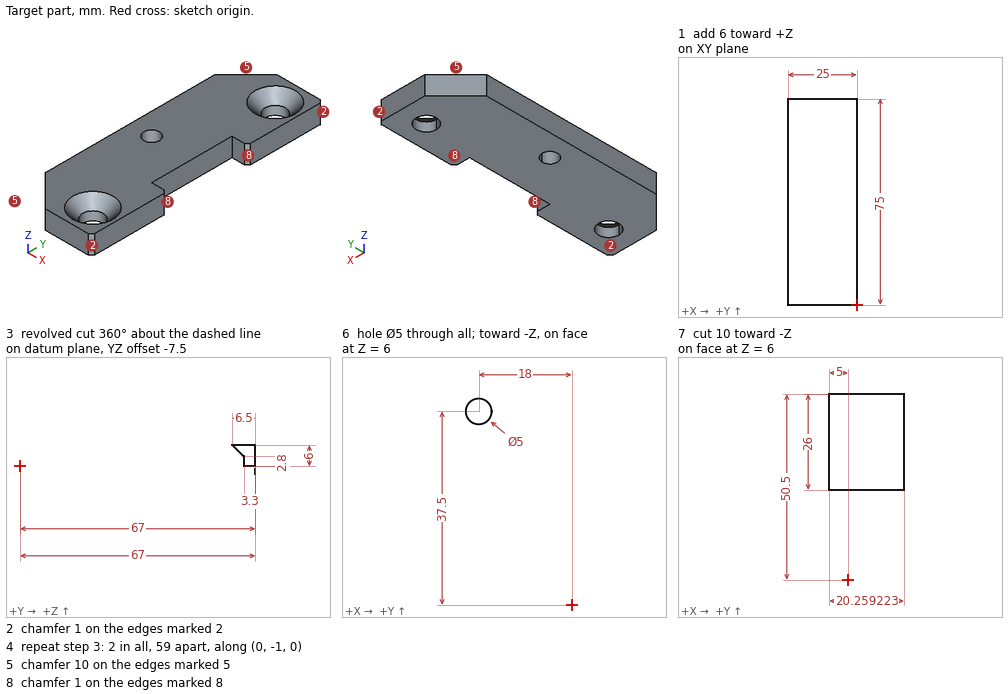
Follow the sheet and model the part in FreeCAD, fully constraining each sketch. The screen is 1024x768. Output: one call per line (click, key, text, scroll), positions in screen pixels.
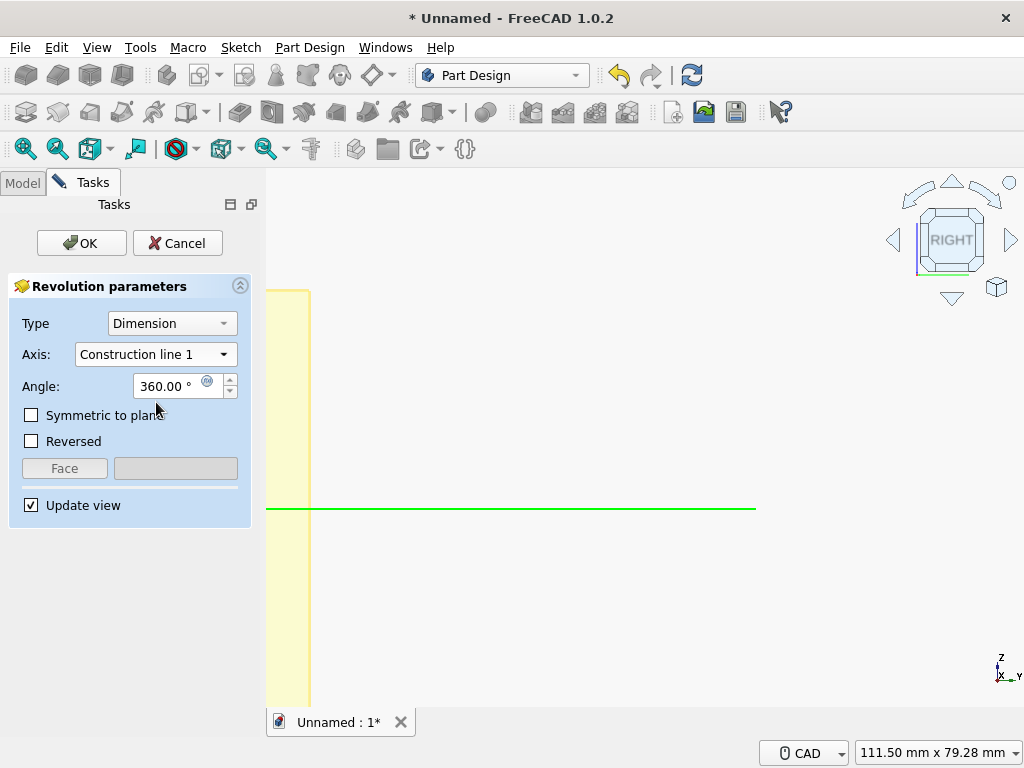
click(82, 243)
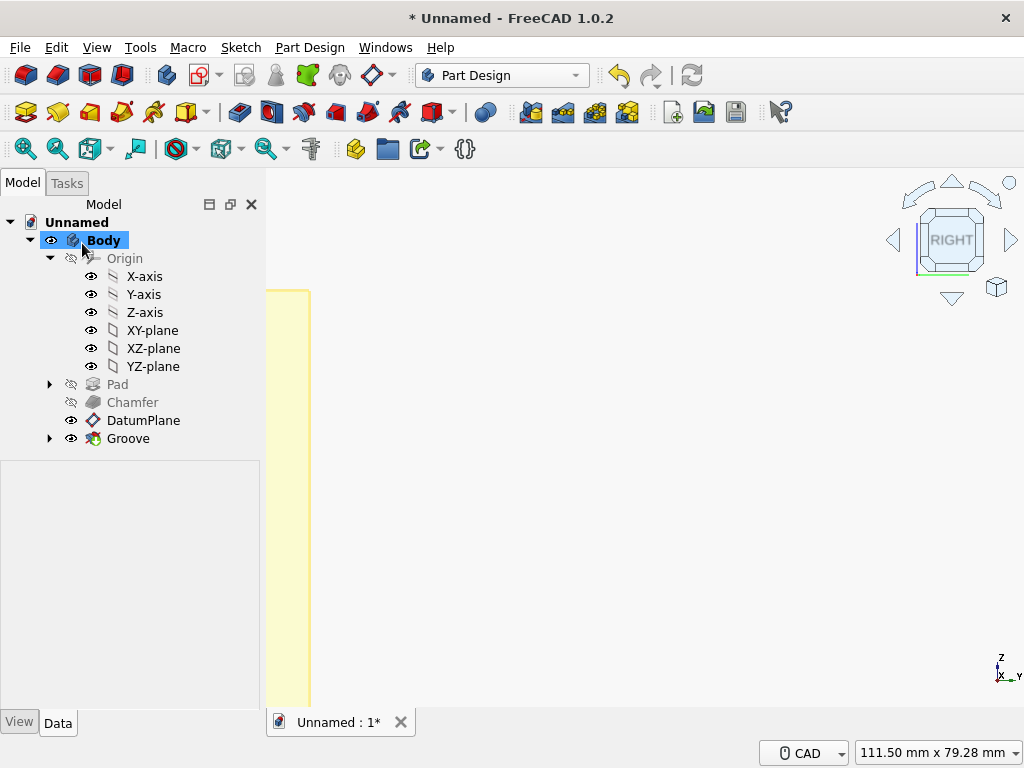
click(116, 420)
key(space)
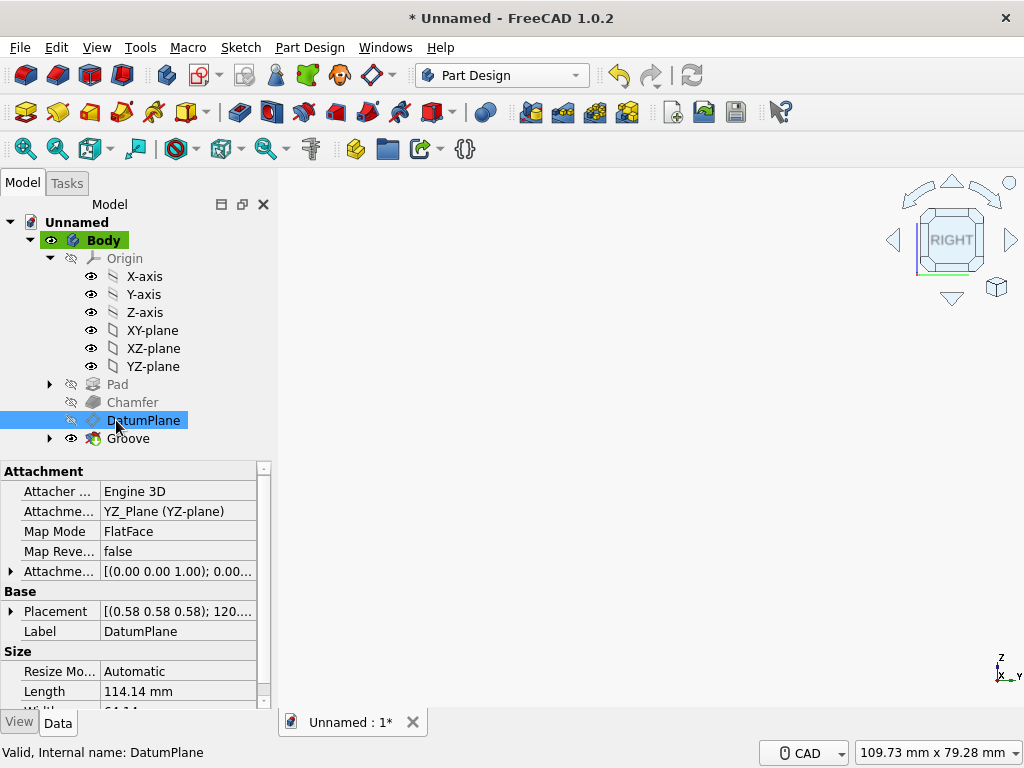
click(26, 150)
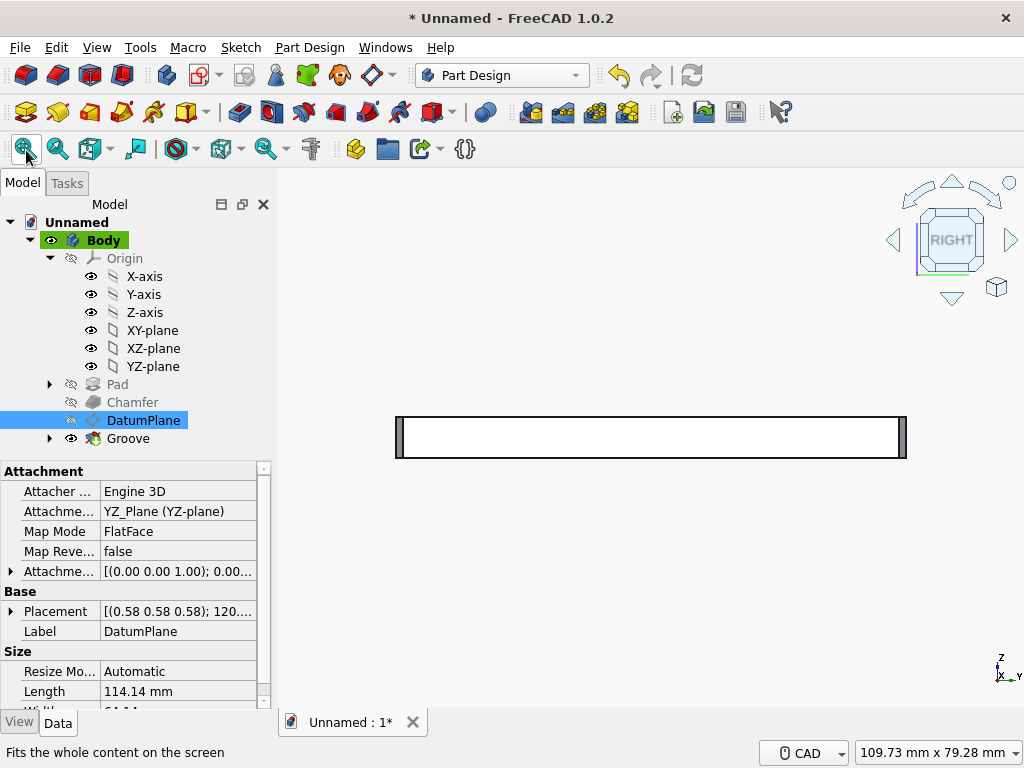
click(116, 438)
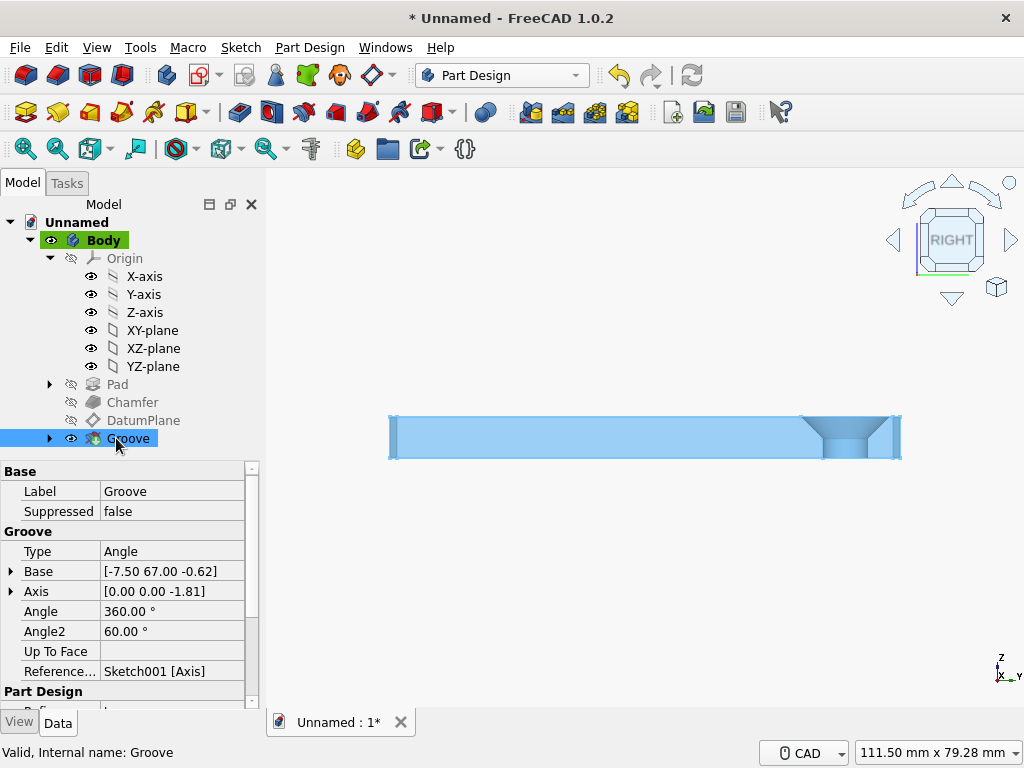
click(564, 112)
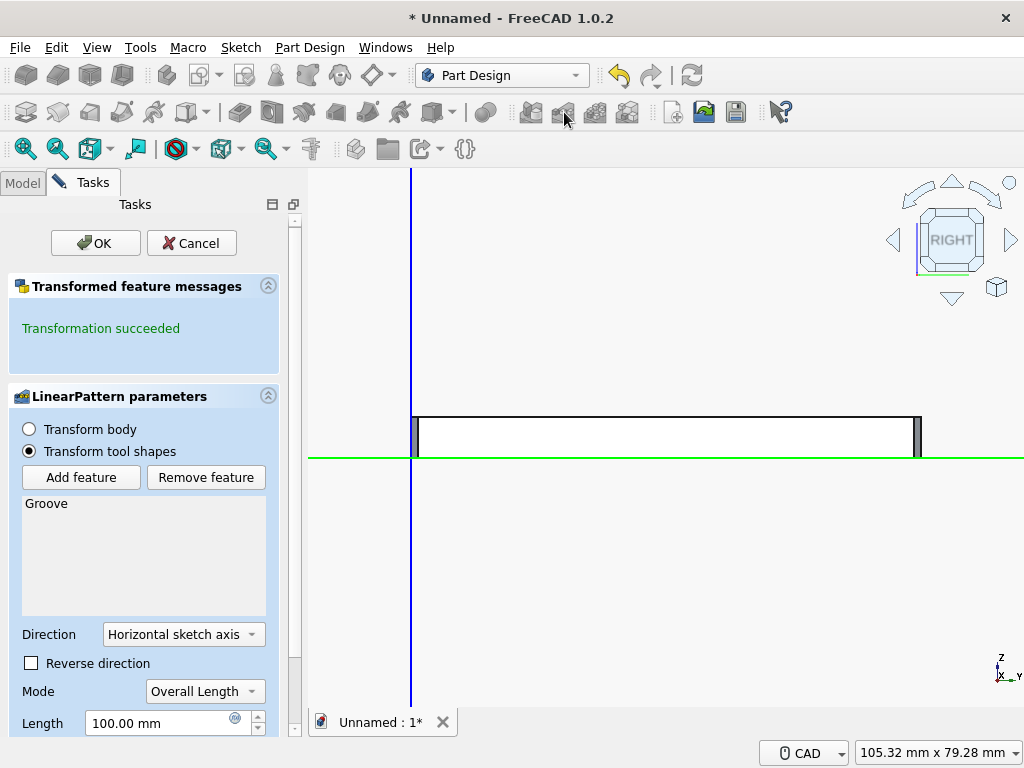
click(184, 634)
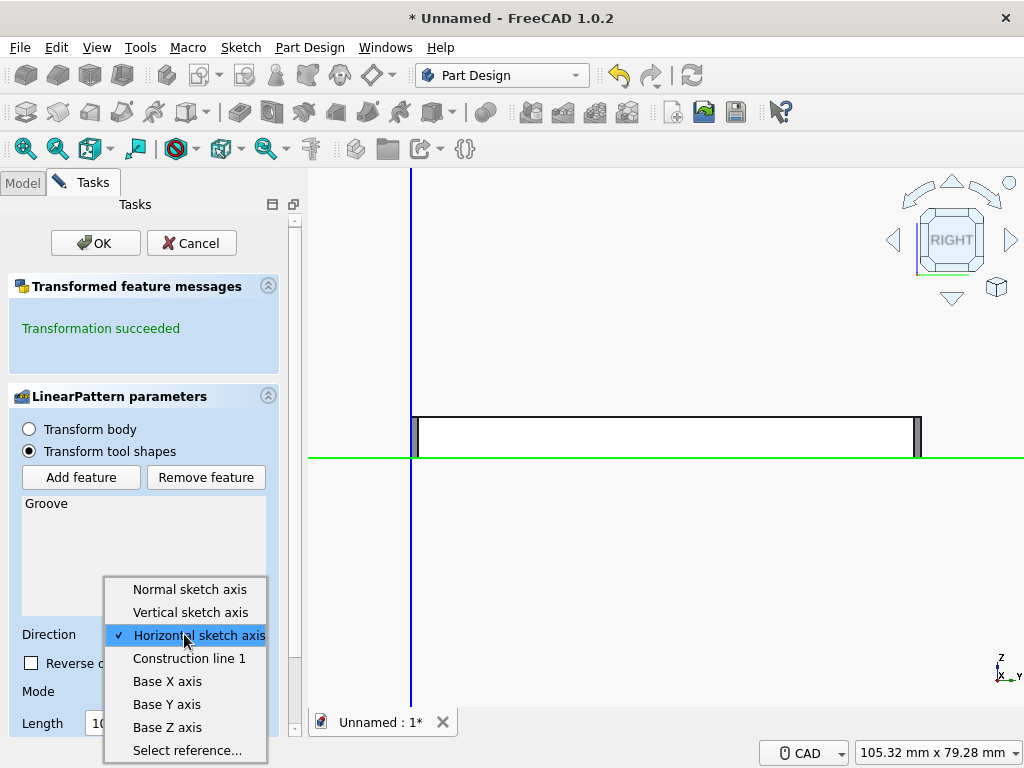
click(184, 704)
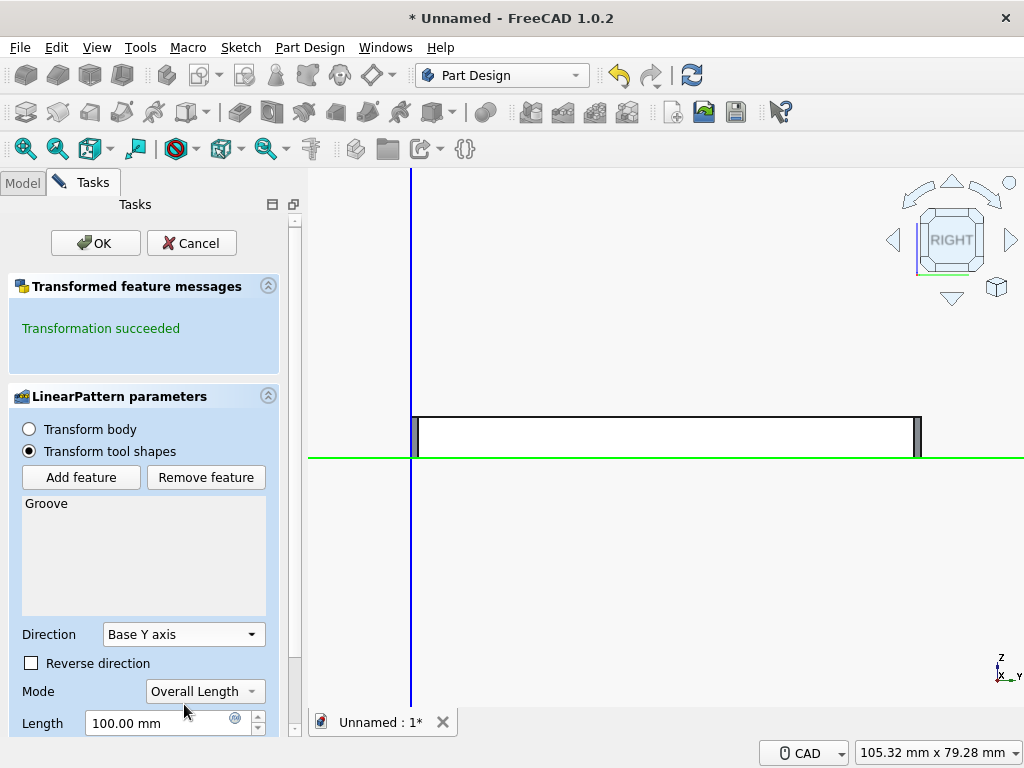
click(206, 692)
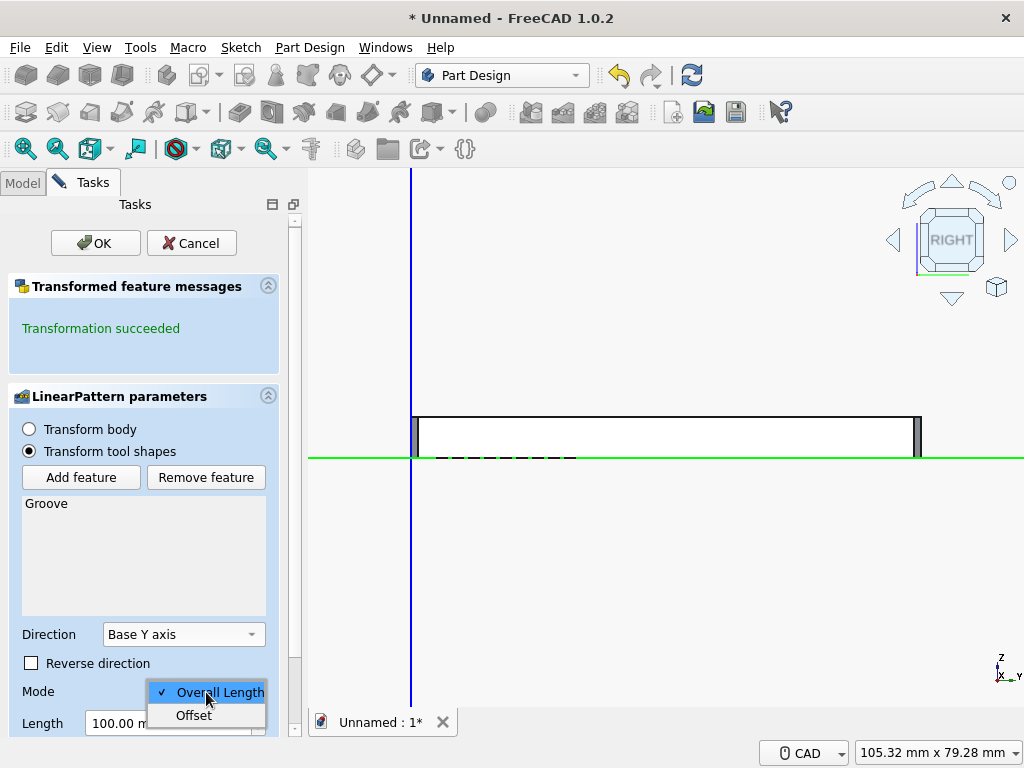
click(206, 716)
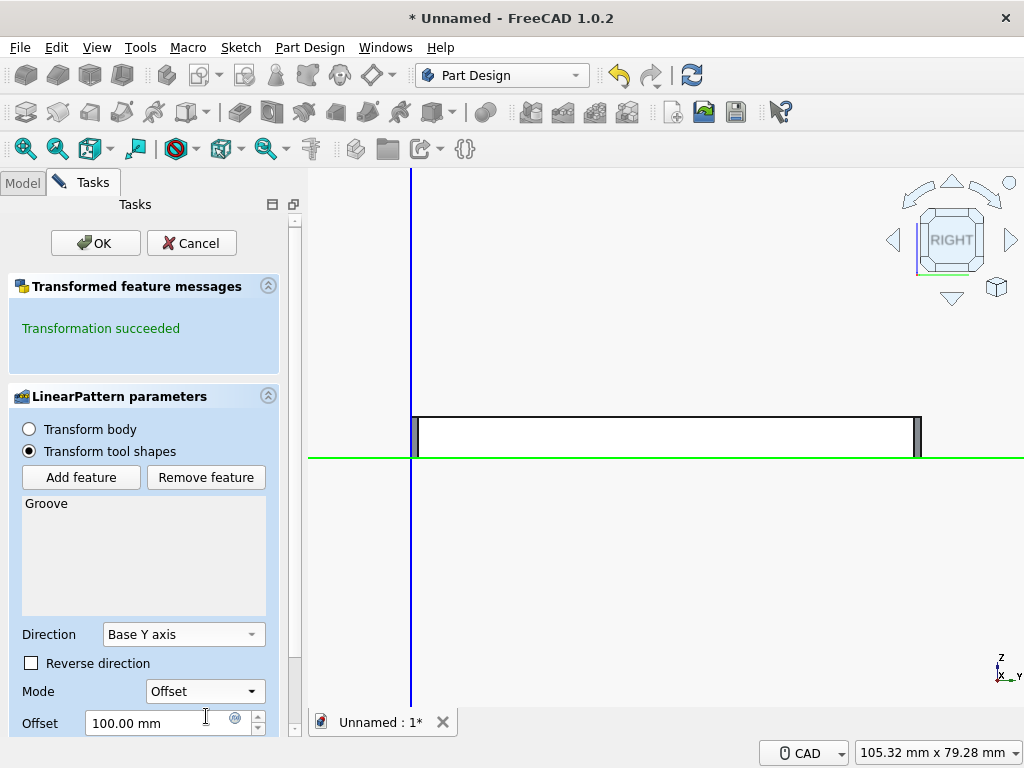
triple_click(168, 723)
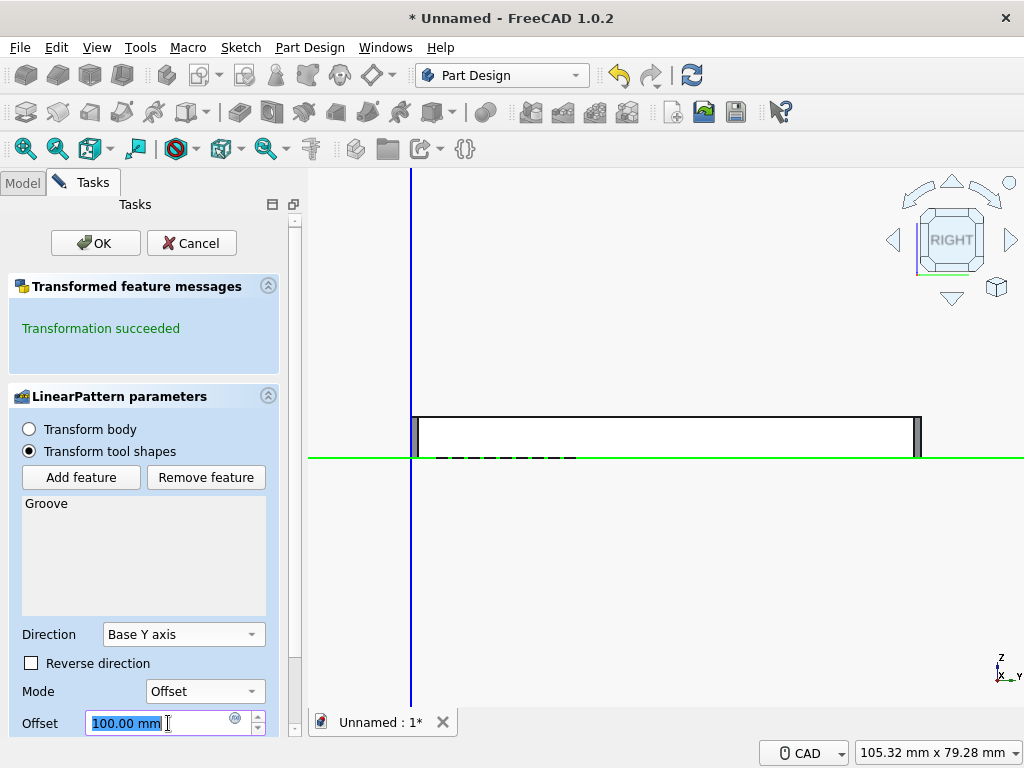
text(59)
key(Tab)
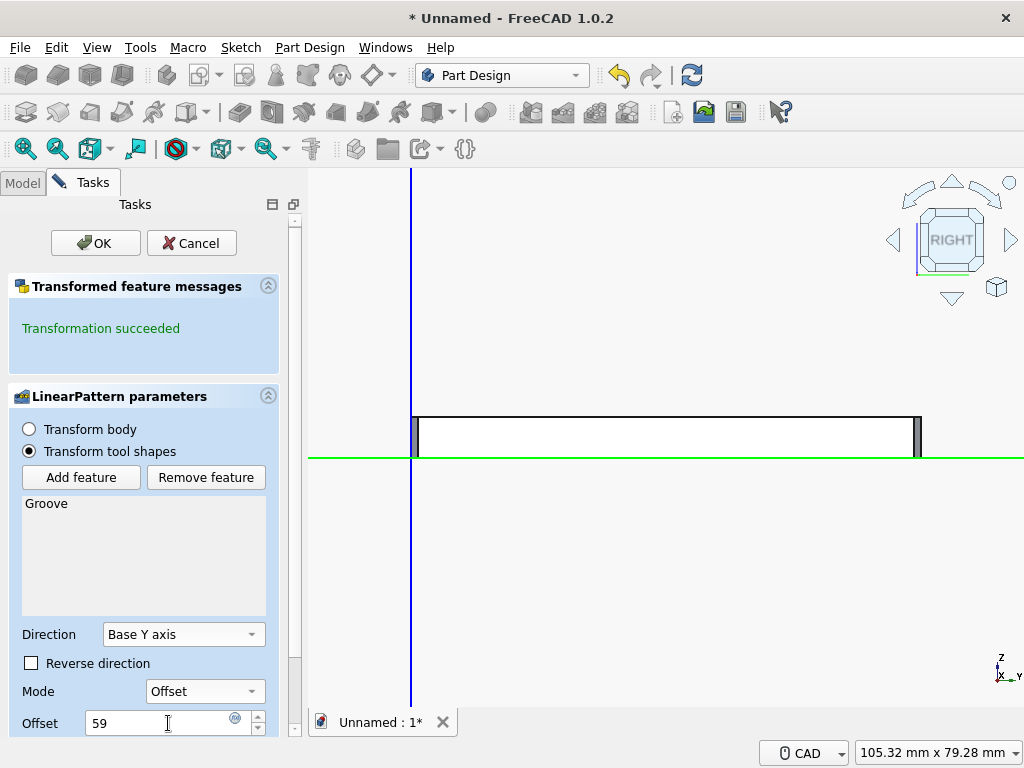
scroll(295, 475, down, 2)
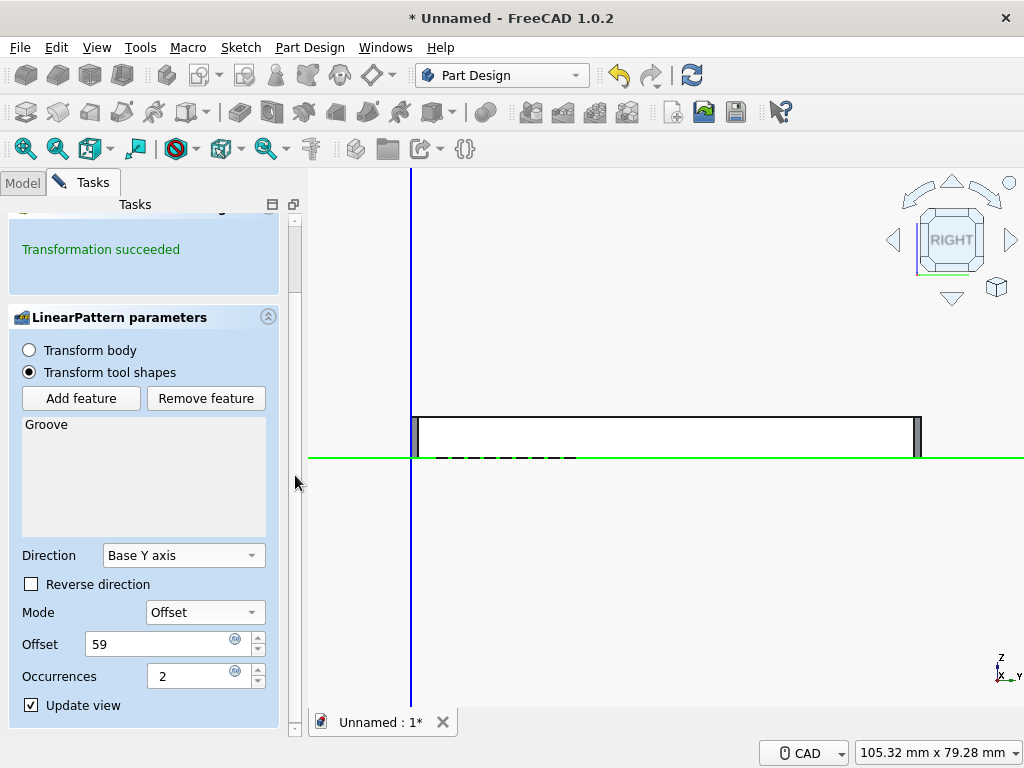
triple_click(198, 676)